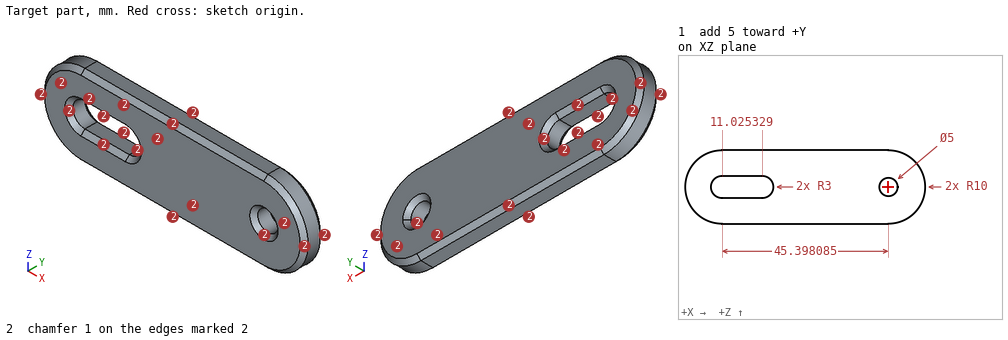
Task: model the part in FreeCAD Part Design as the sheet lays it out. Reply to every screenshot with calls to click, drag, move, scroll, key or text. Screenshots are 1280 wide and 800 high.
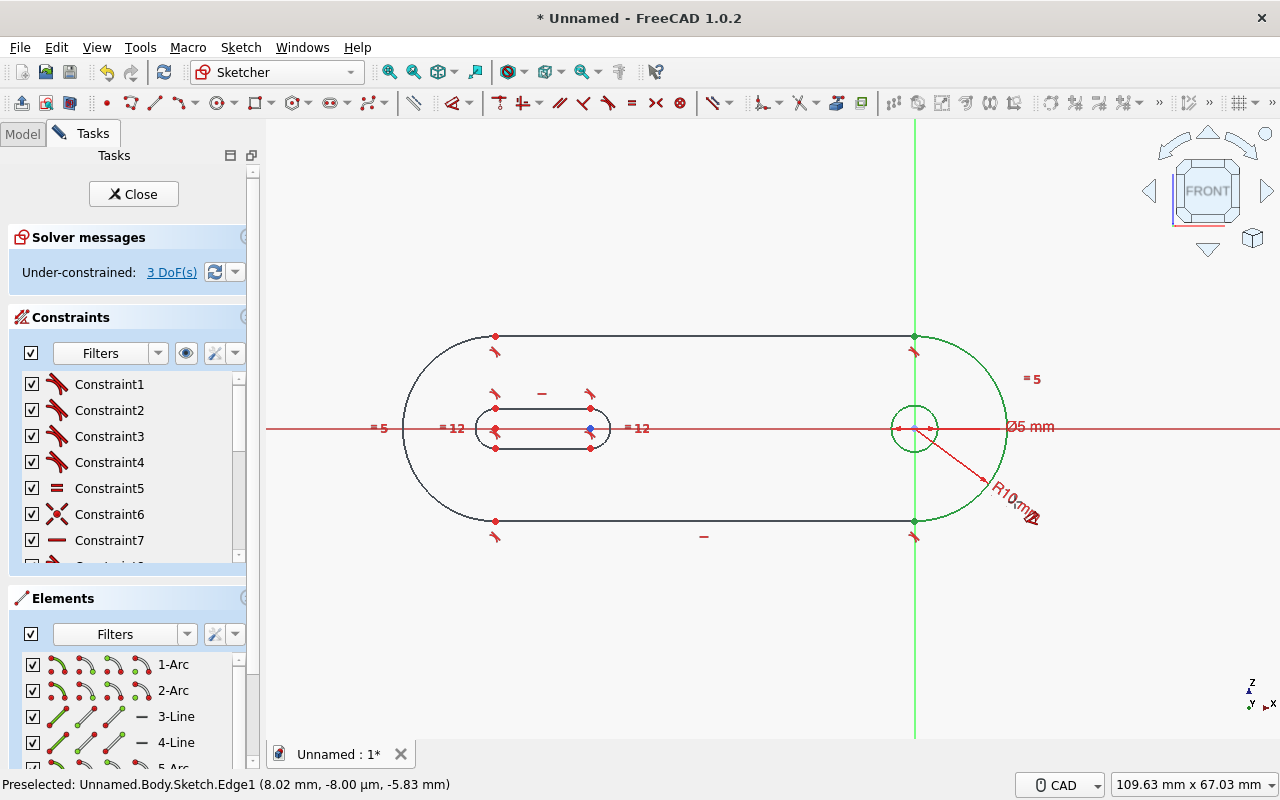
scroll(479, 417, up, 2)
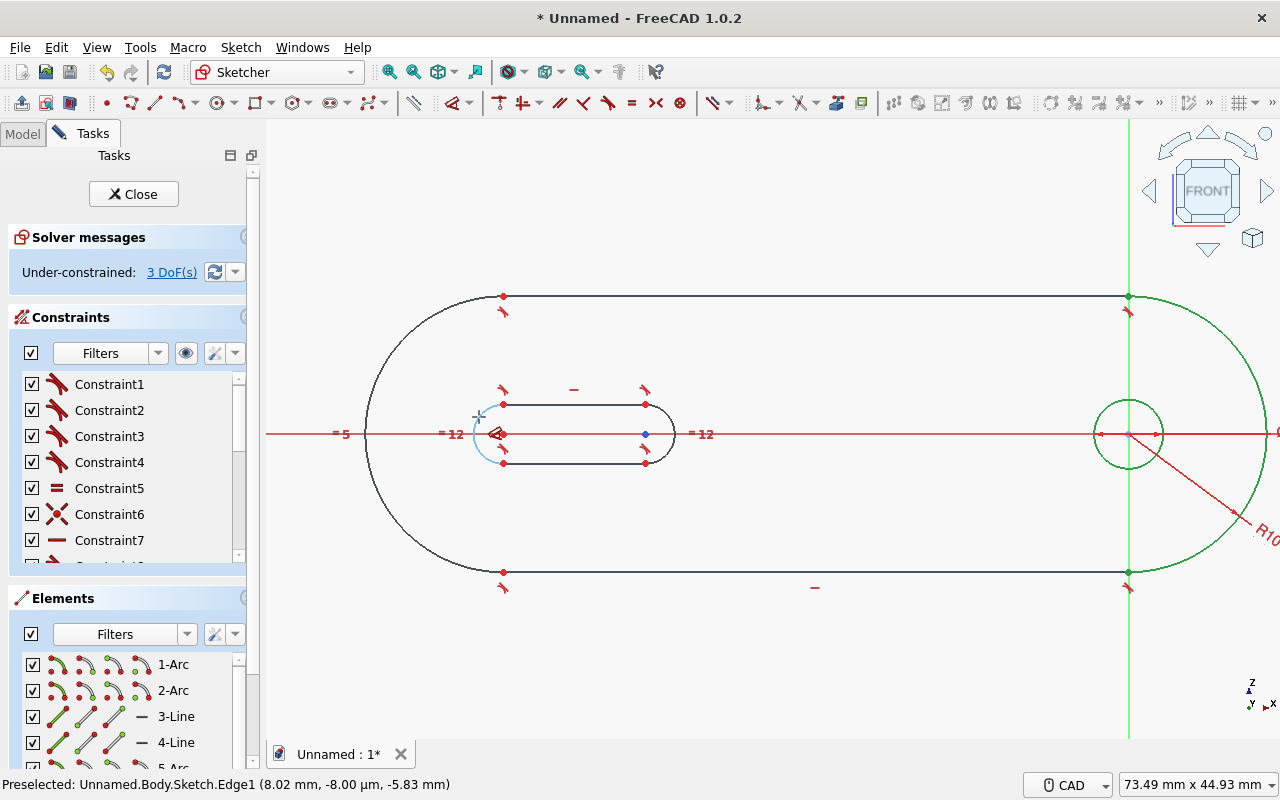
click(479, 417)
click(453, 398)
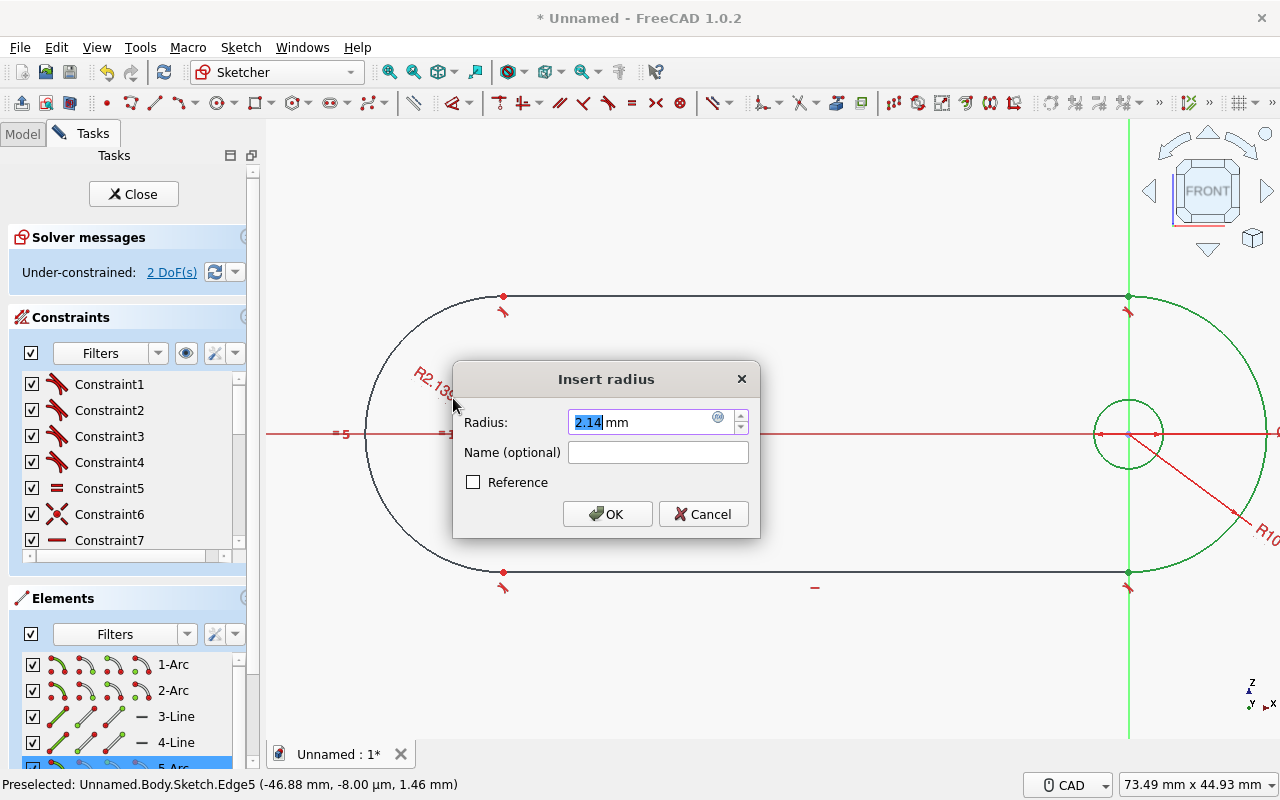
text(3)
key(Return)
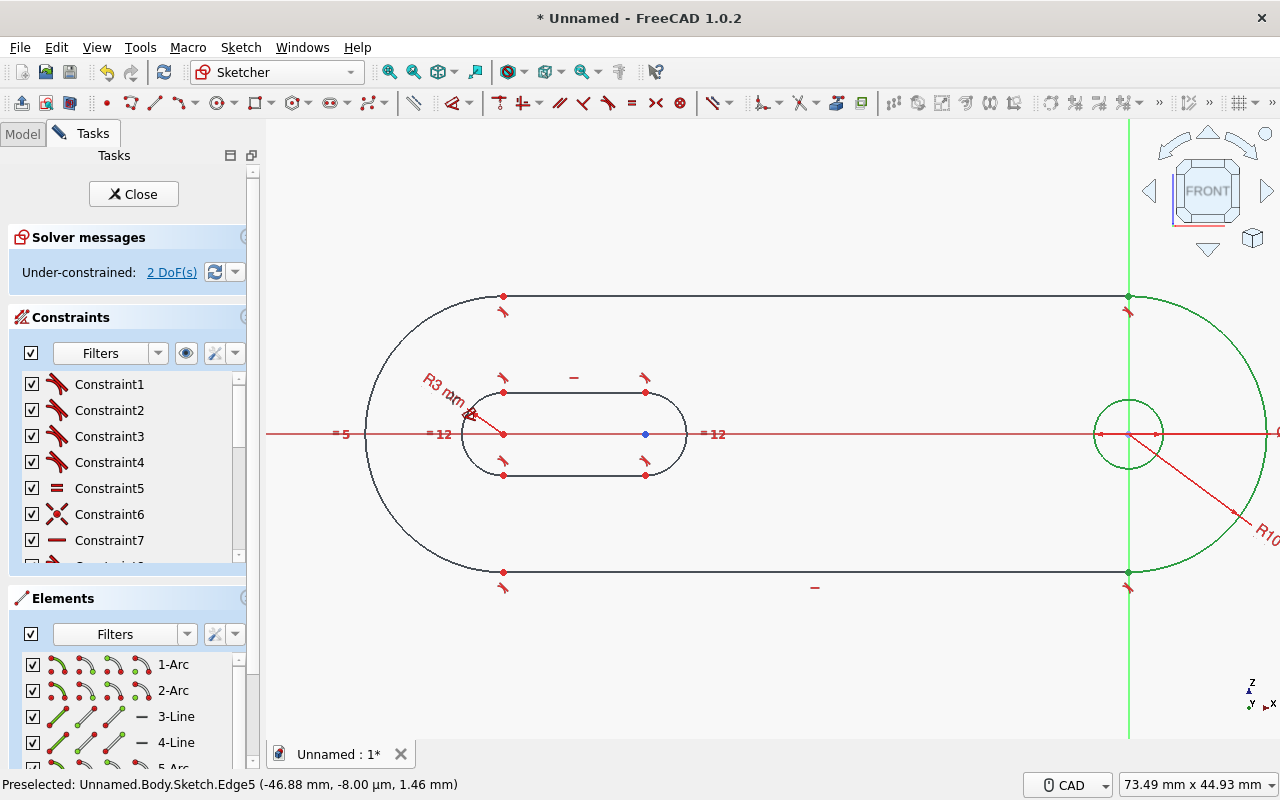
click(941, 572)
click(809, 606)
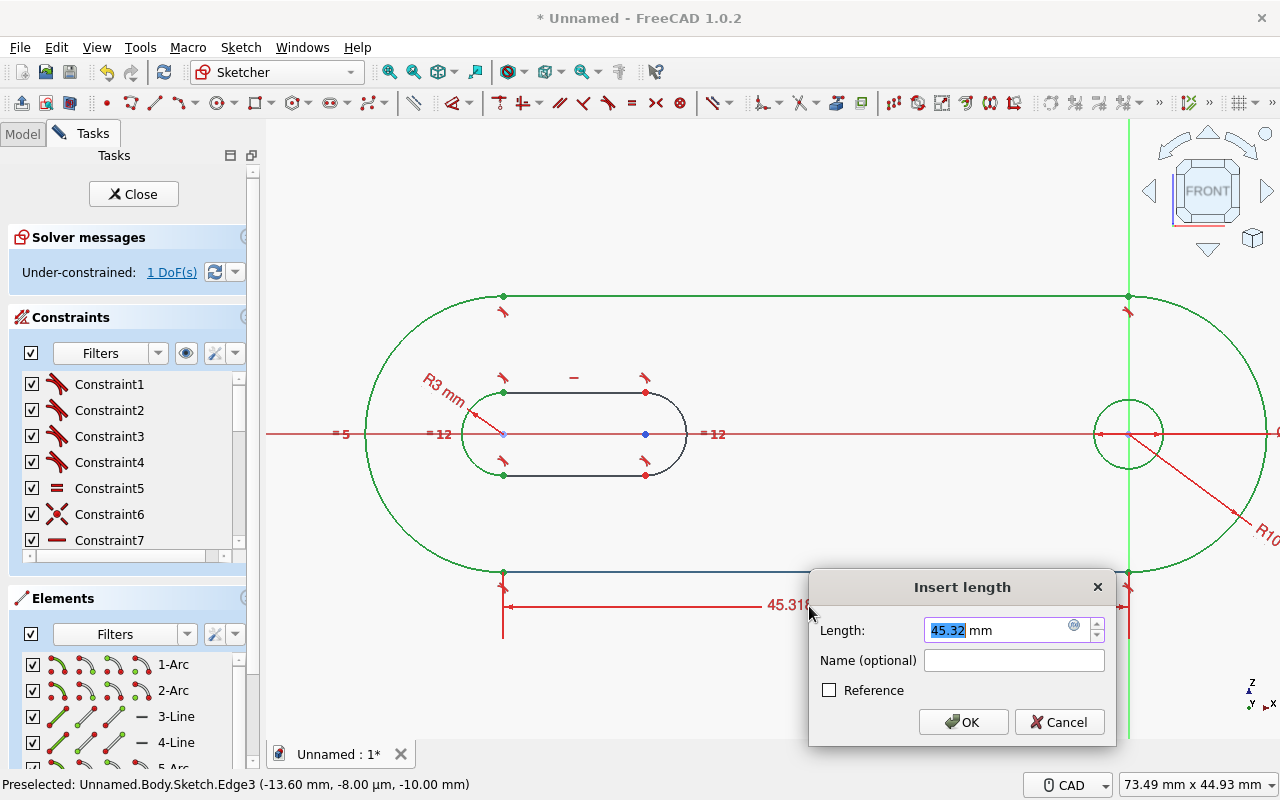
text(45.398085)
key(Return)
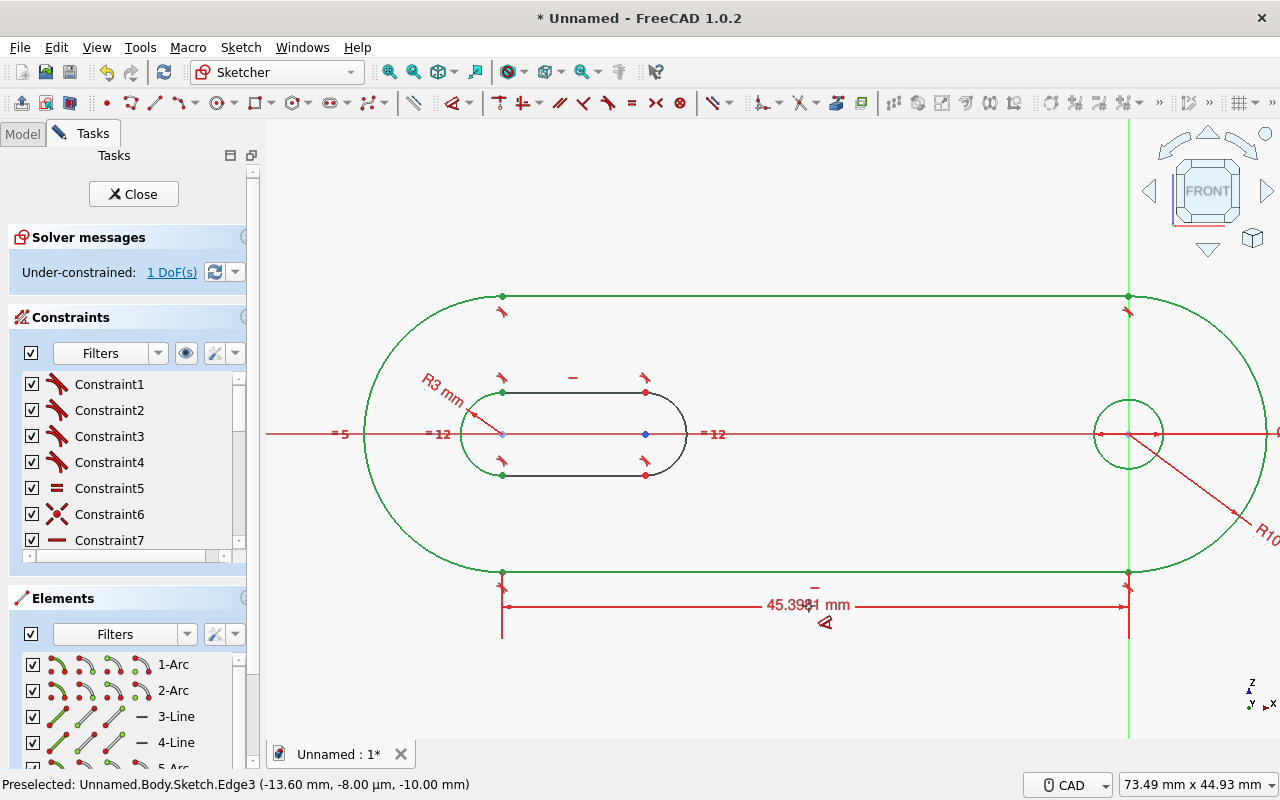
click(545, 393)
click(574, 359)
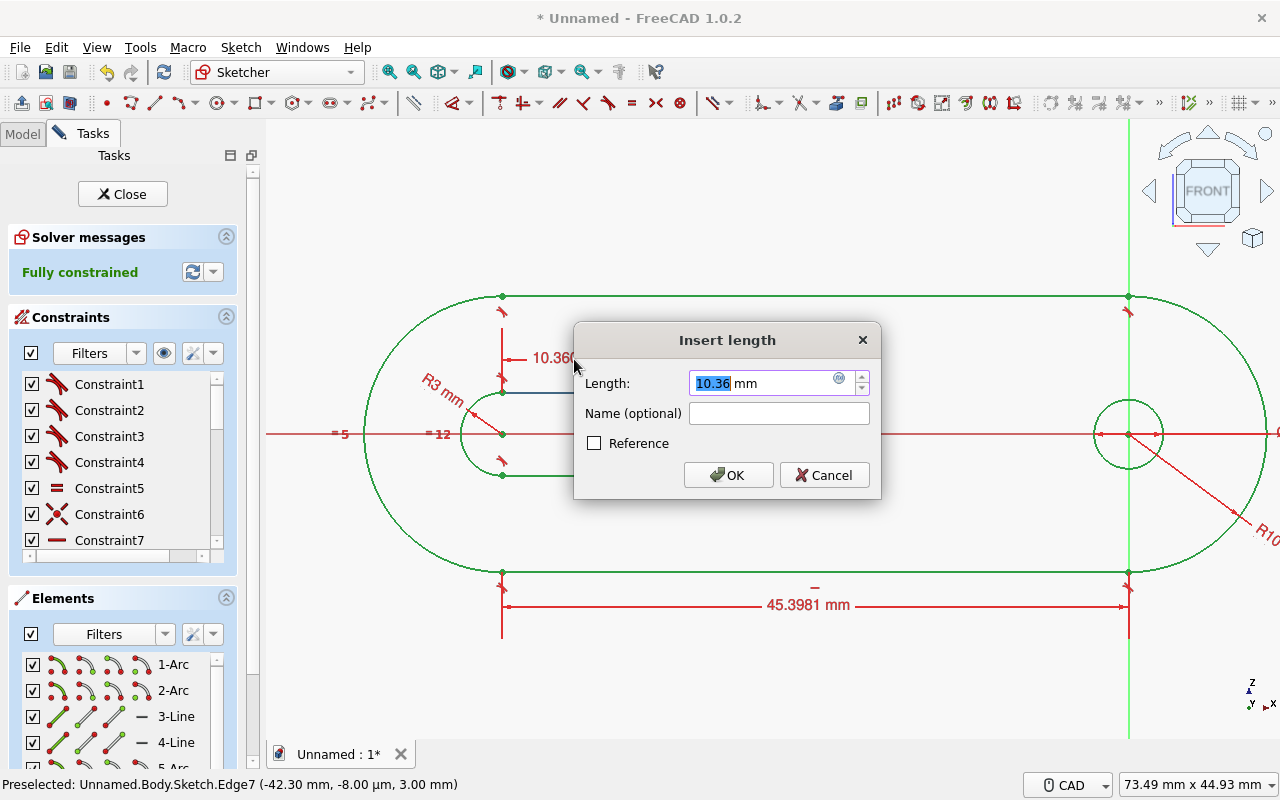
text(11.025329)
key(Return)
key(Escape)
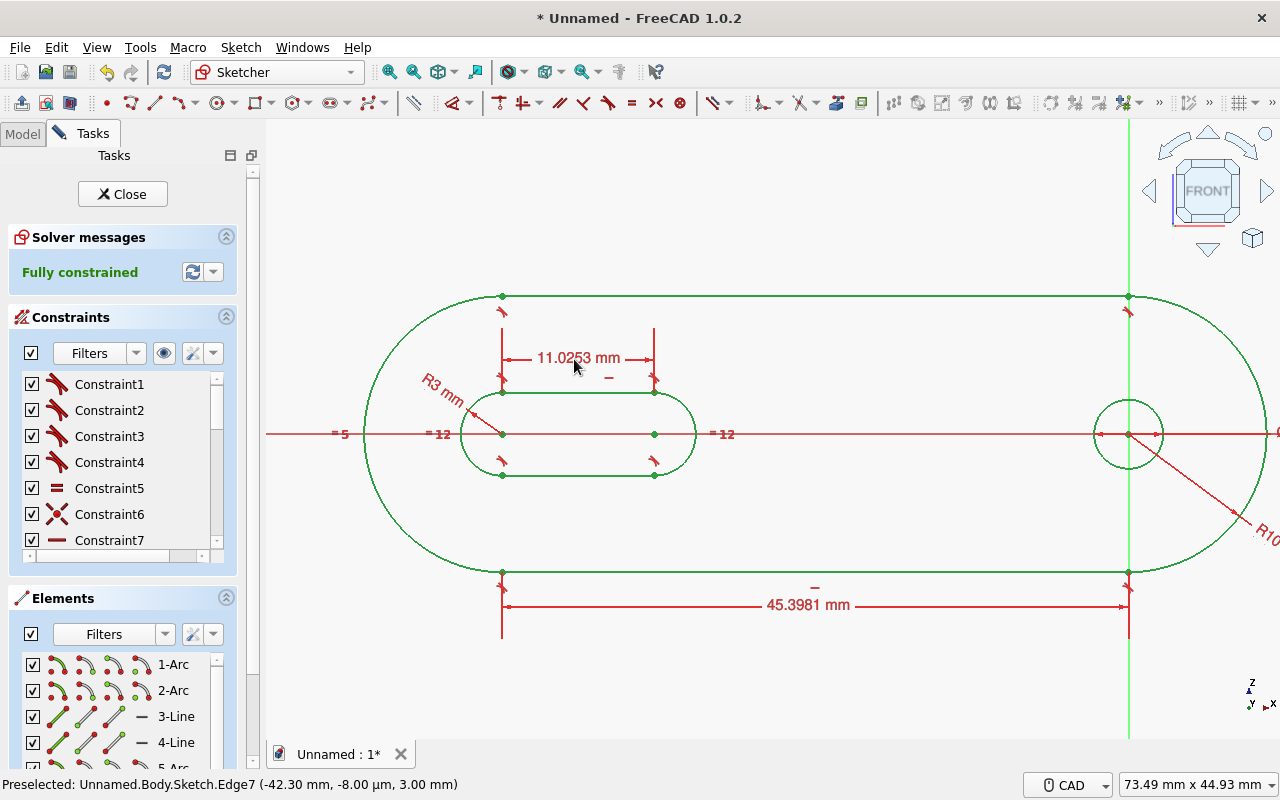
click(123, 194)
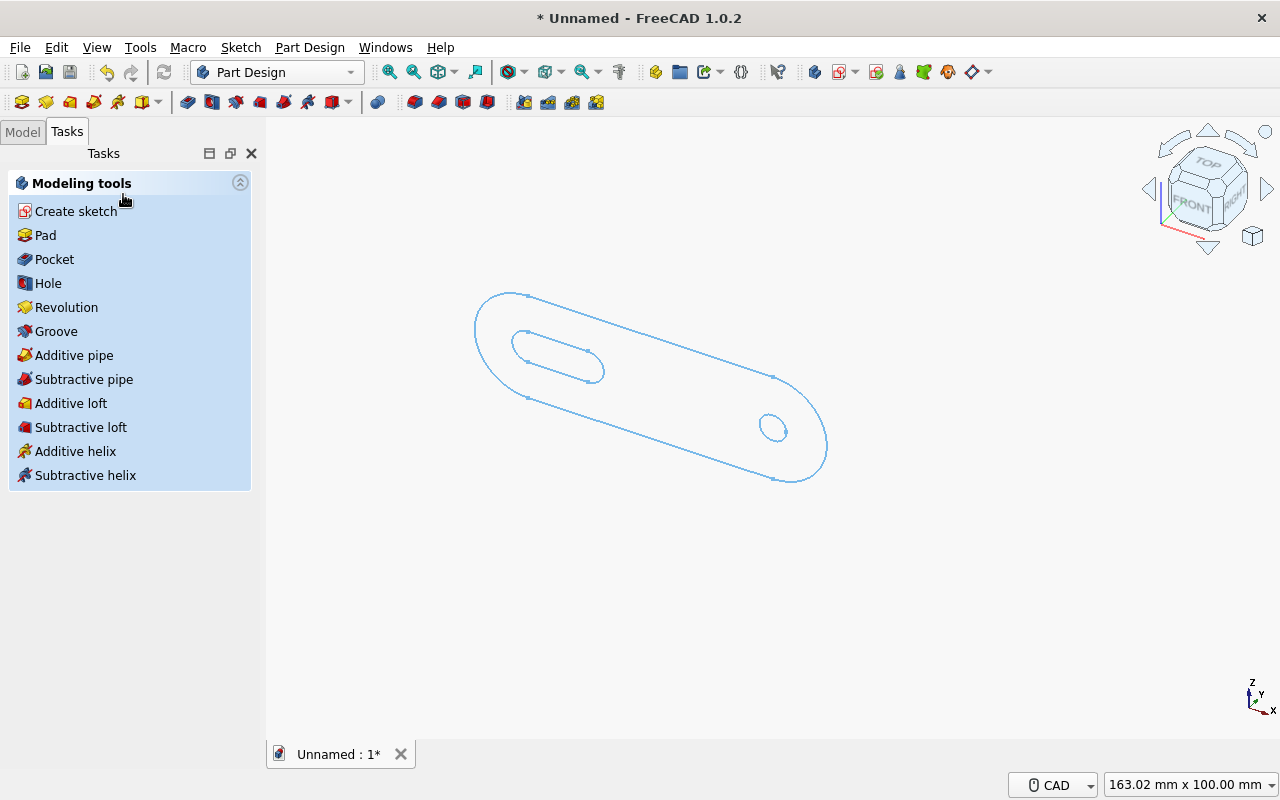
click(22, 102)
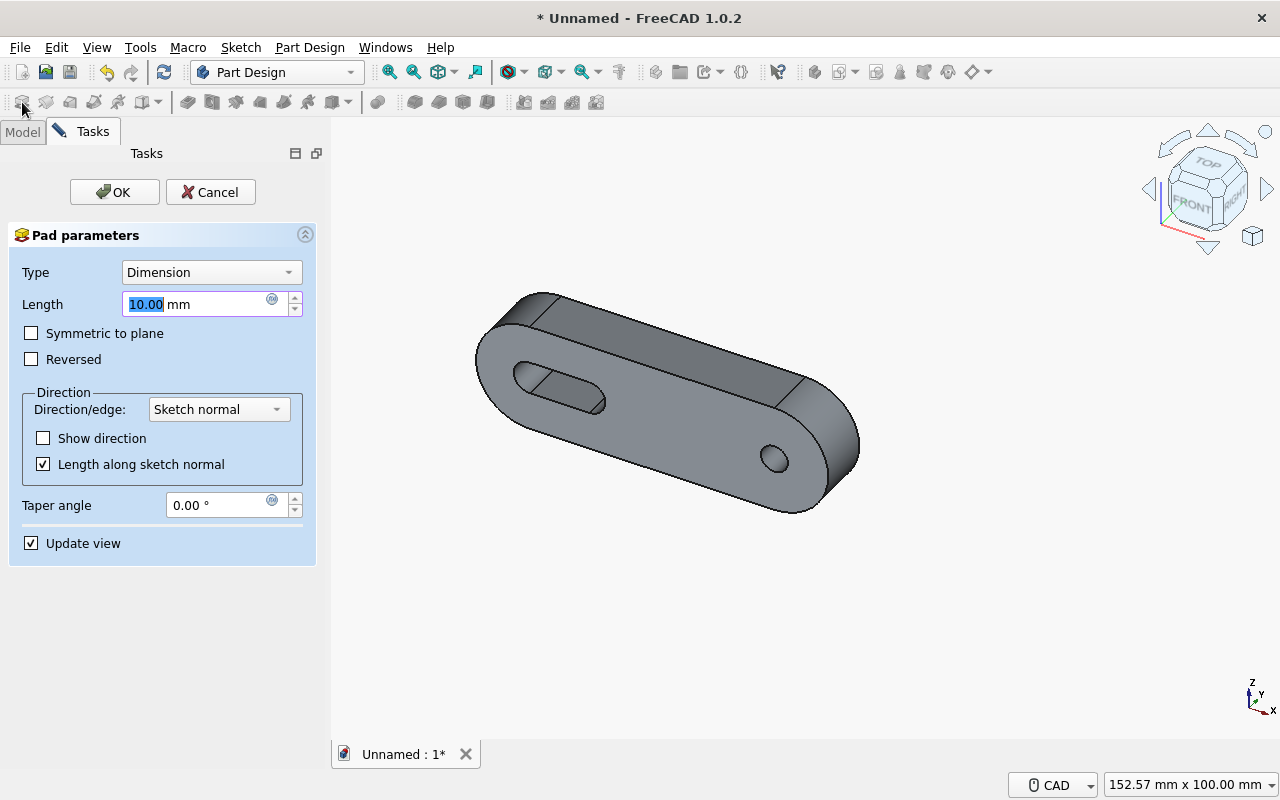
text(5)
key(Tab)